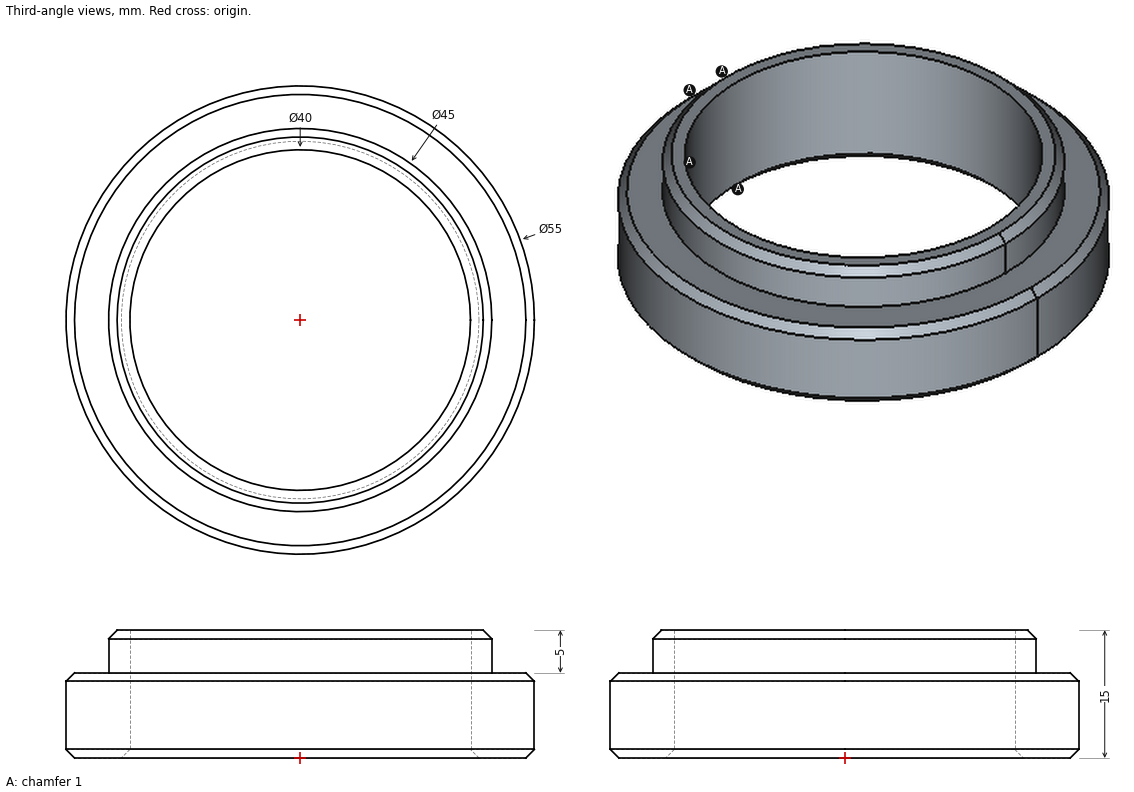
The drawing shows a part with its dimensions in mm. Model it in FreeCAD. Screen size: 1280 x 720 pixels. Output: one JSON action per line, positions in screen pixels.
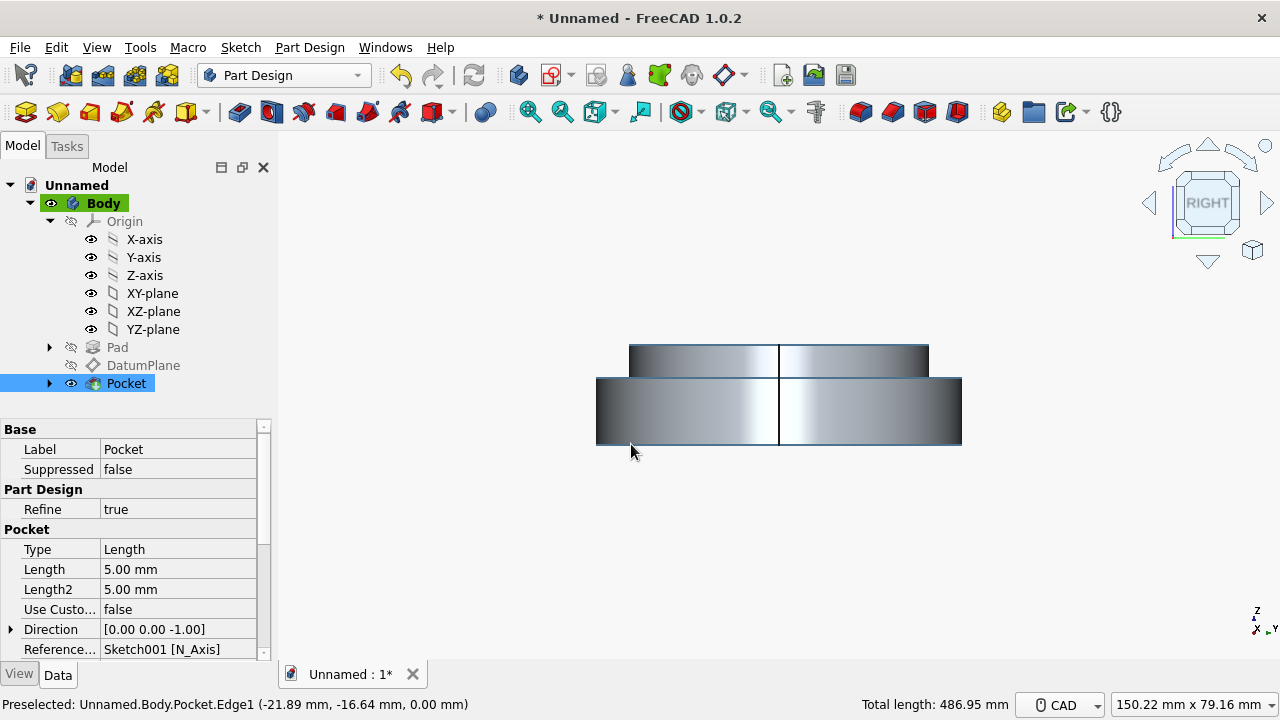
{"action": "key", "text": "v f"}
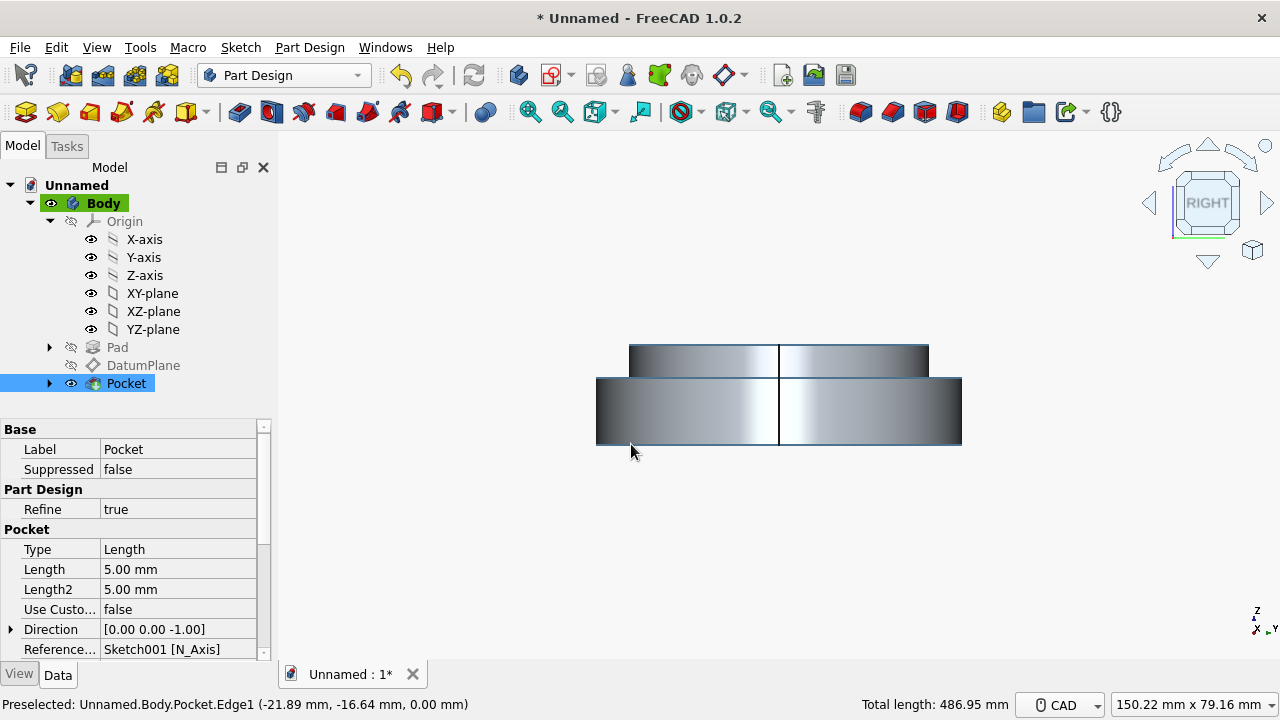
{"action": "key", "text": "5"}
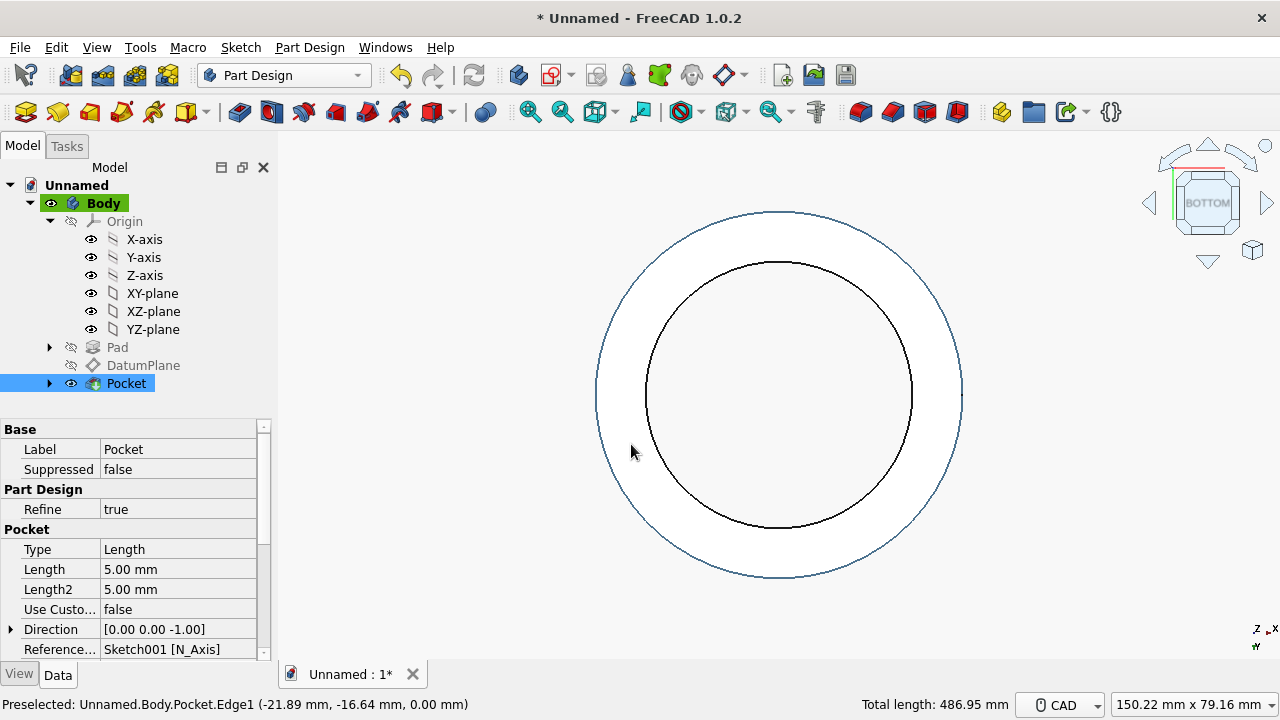
{"action": "left_click", "coordinate": [646, 394], "text": "ctrl"}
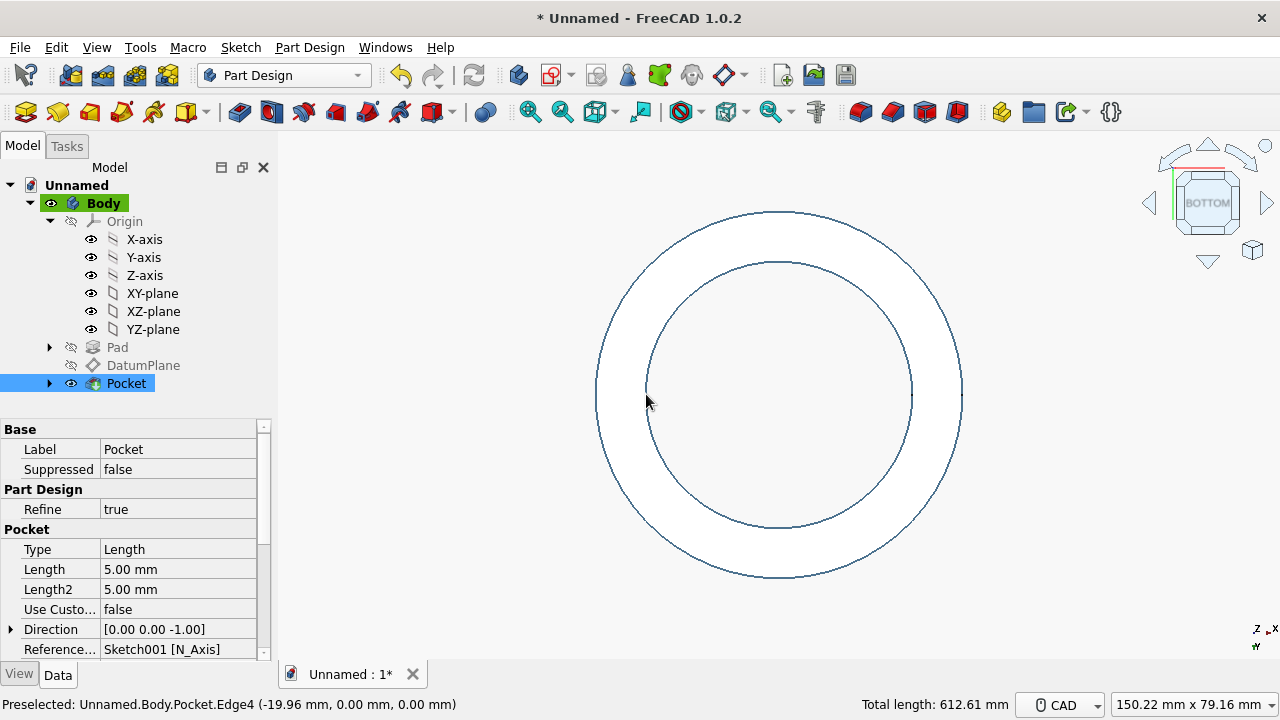
{"action": "left_click", "coordinate": [894, 112]}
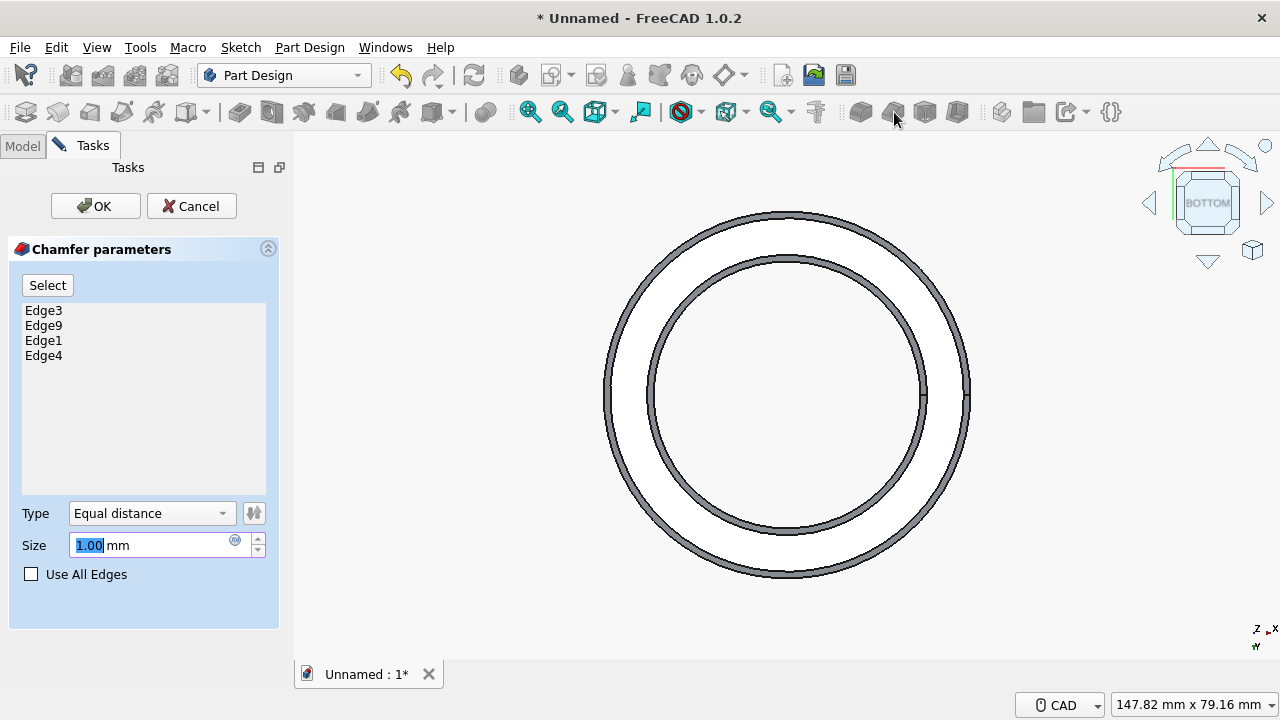
{"action": "type", "text": "1"}
{"action": "key", "text": "Tab"}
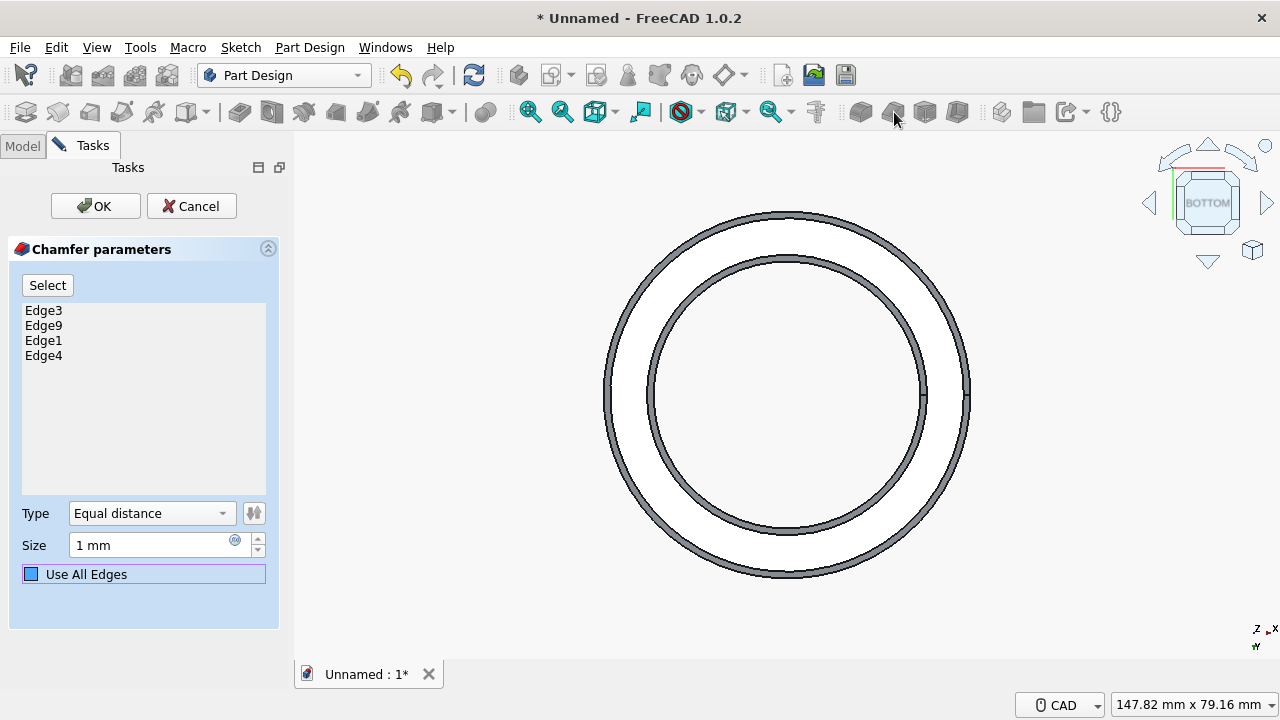
{"action": "left_click", "coordinate": [96, 206]}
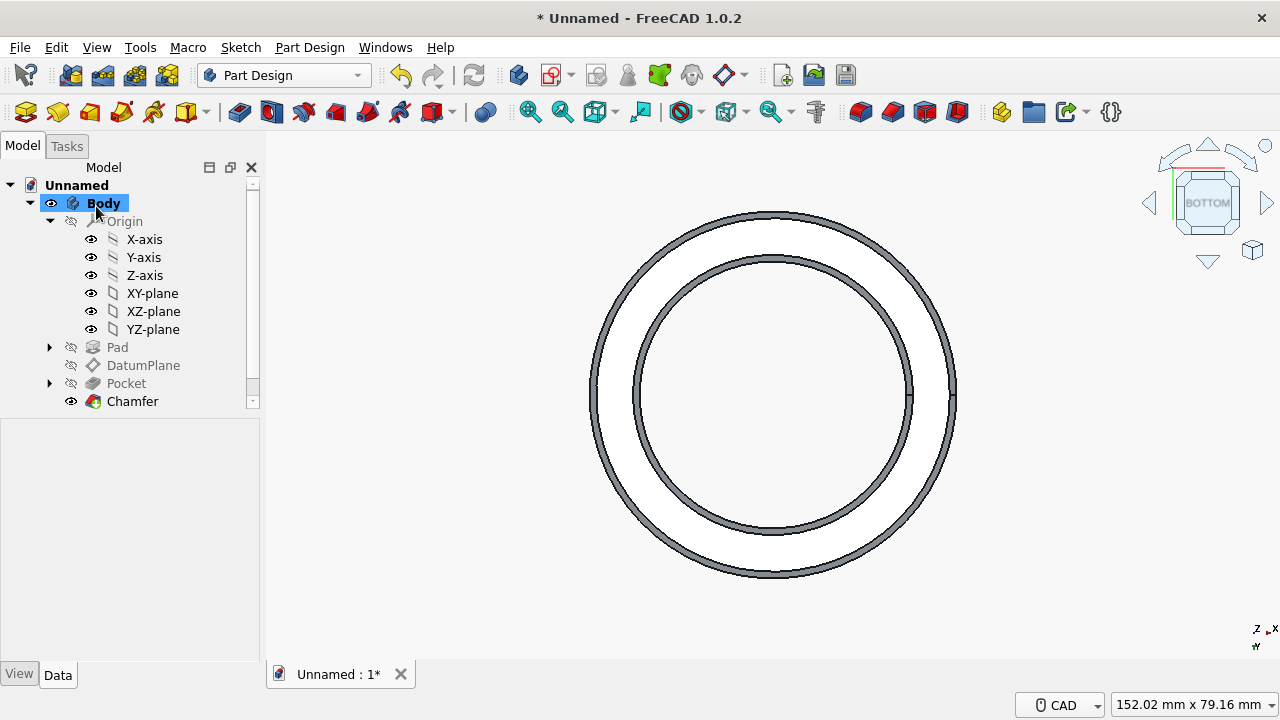
{"action": "key", "text": "0"}